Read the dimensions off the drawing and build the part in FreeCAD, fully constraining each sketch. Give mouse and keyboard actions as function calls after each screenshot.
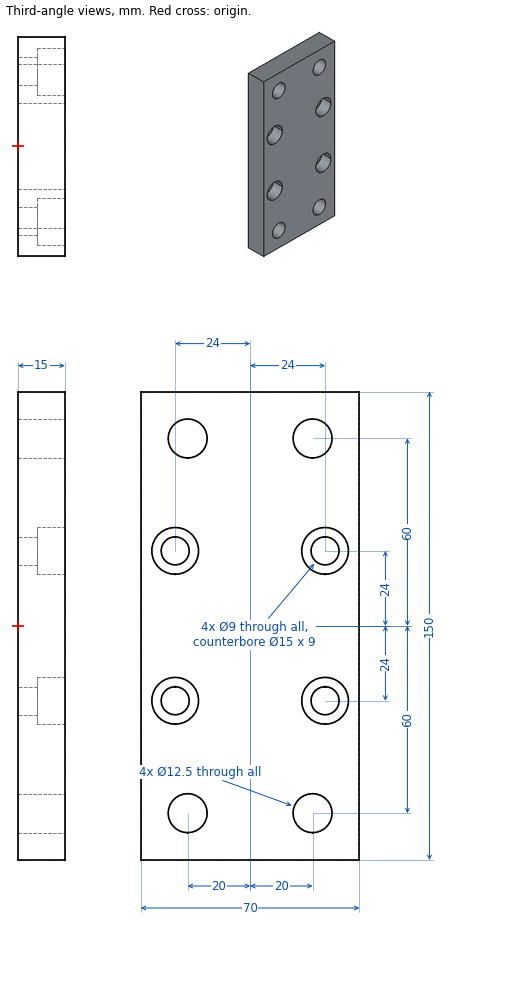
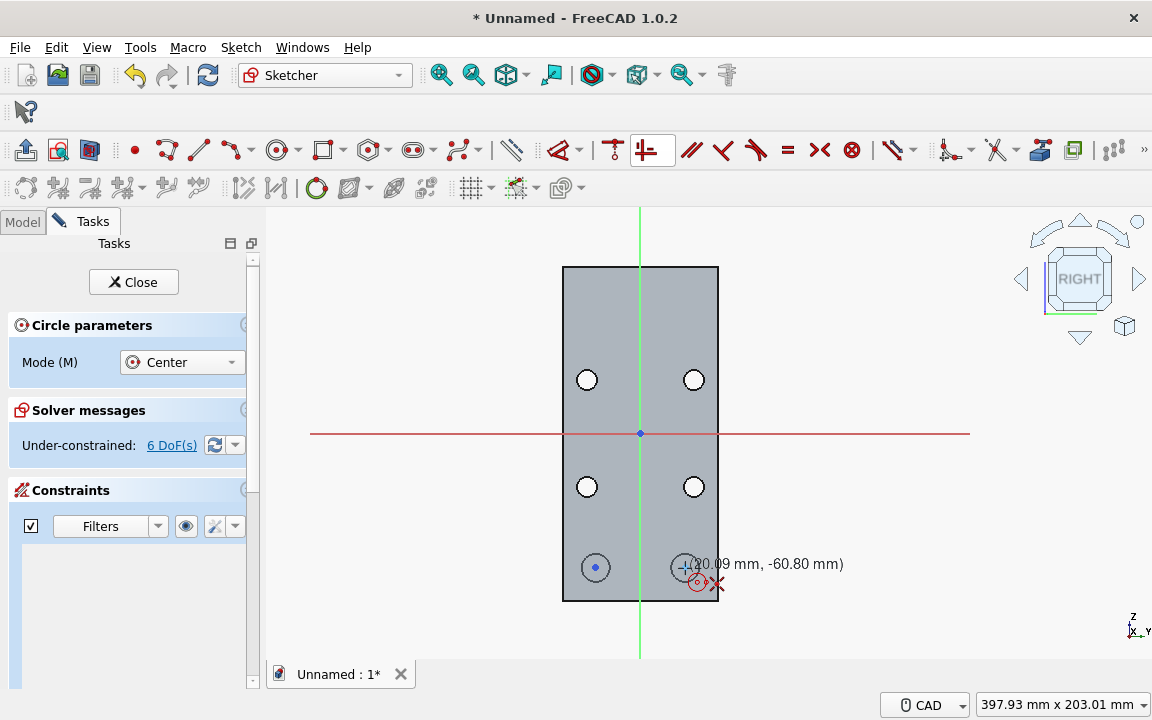
scroll(685, 300, up, 3)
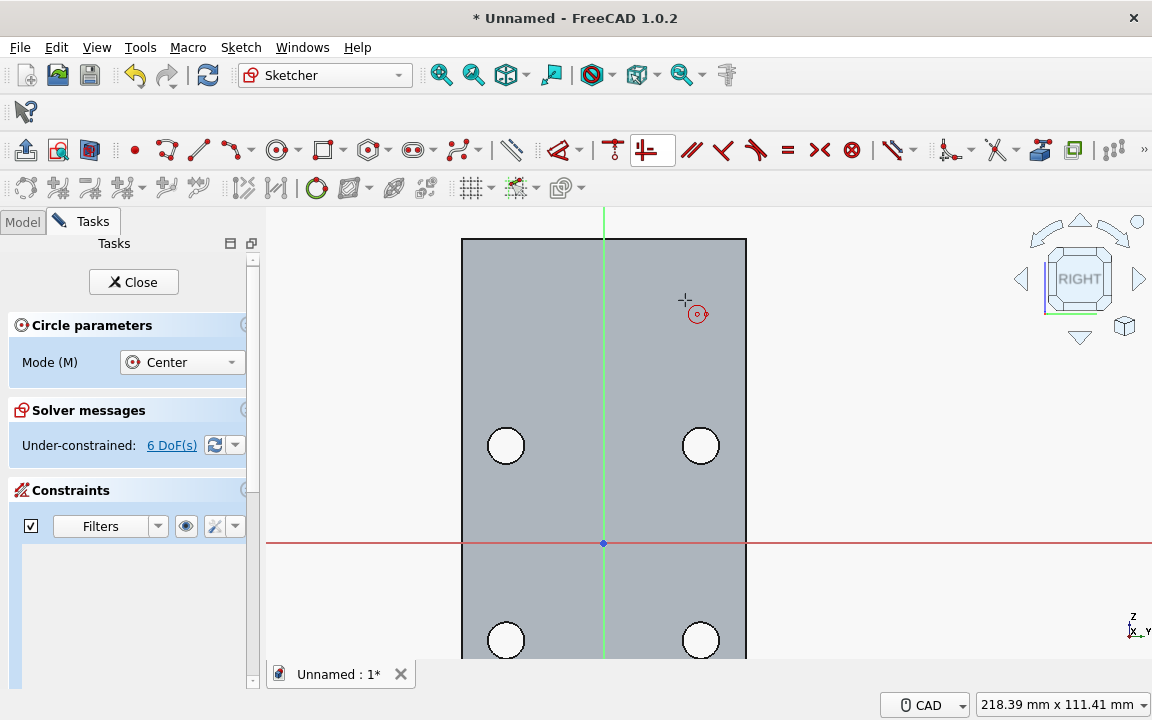
click(685, 300)
click(703, 282)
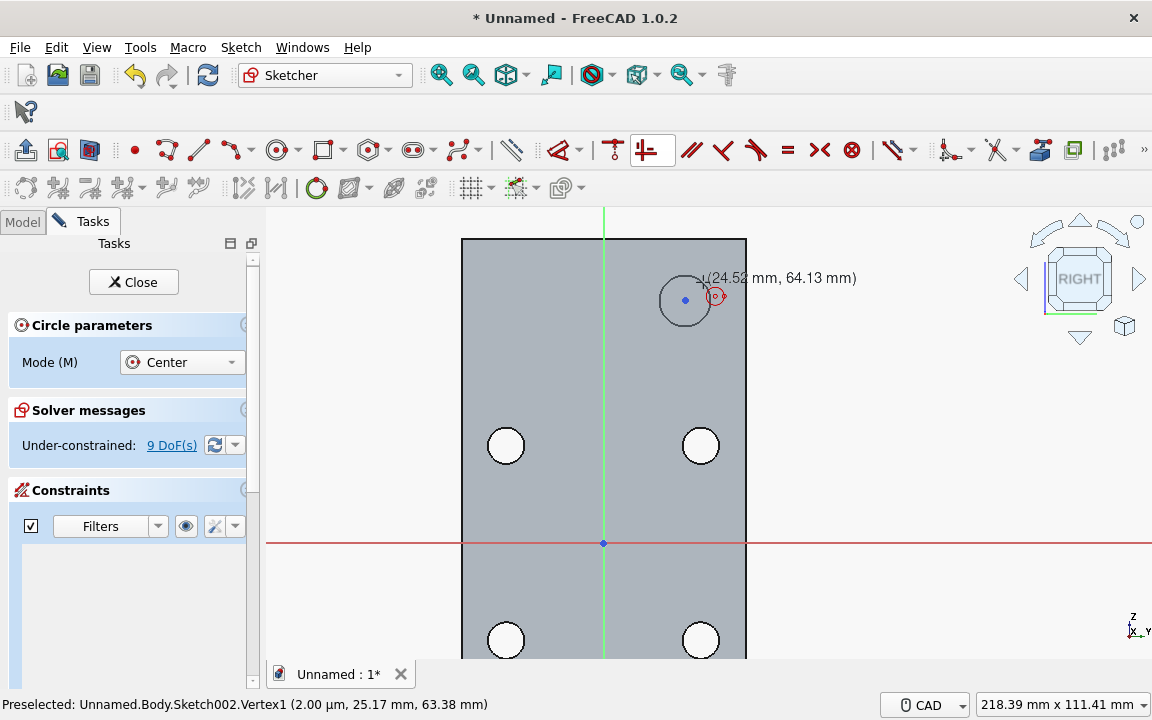
click(522, 300)
click(540, 282)
key(Escape)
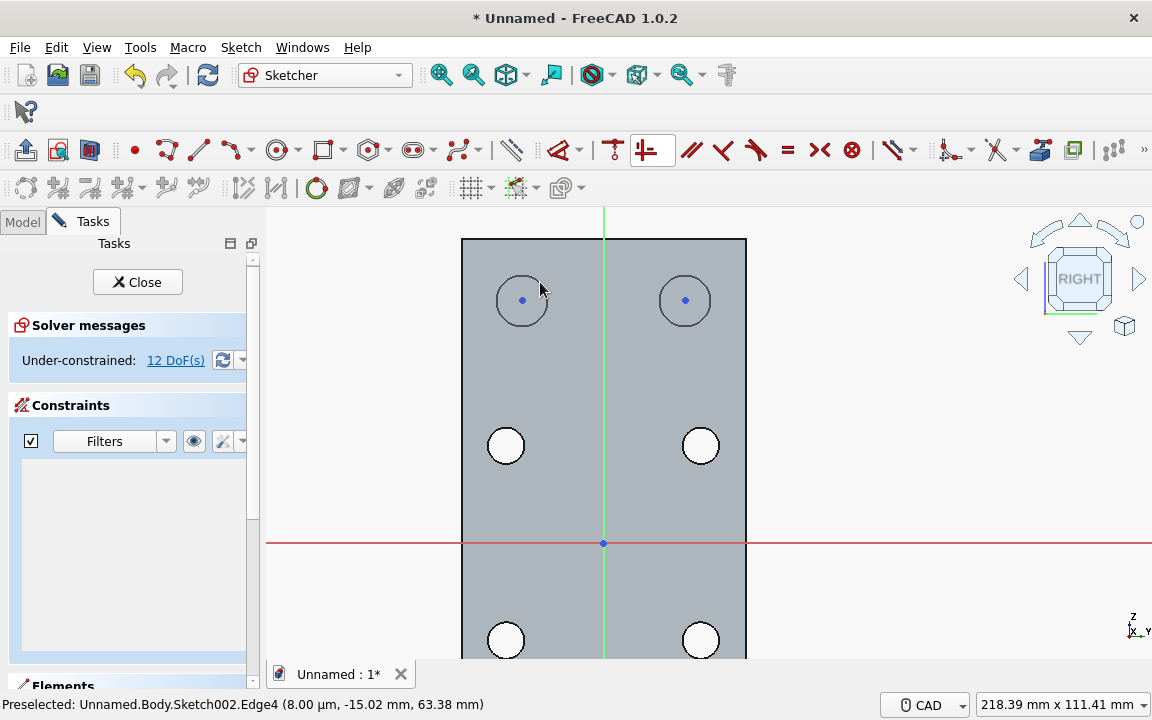
scroll(685, 299, down, 3)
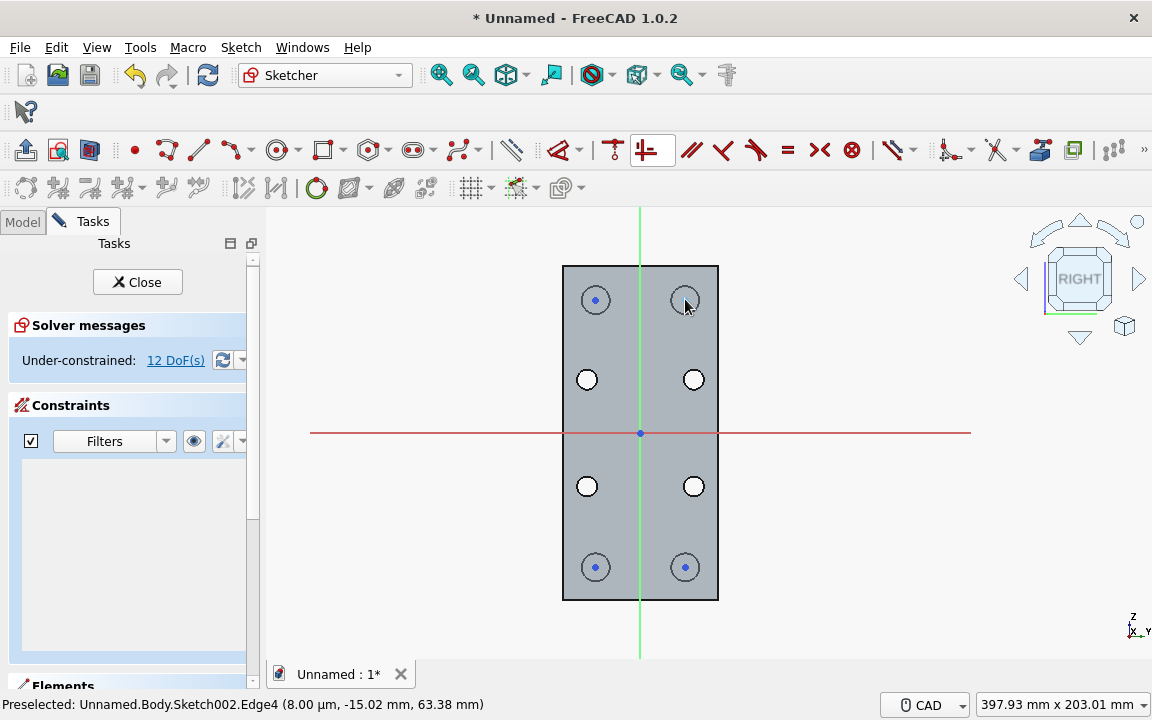
click(695, 557)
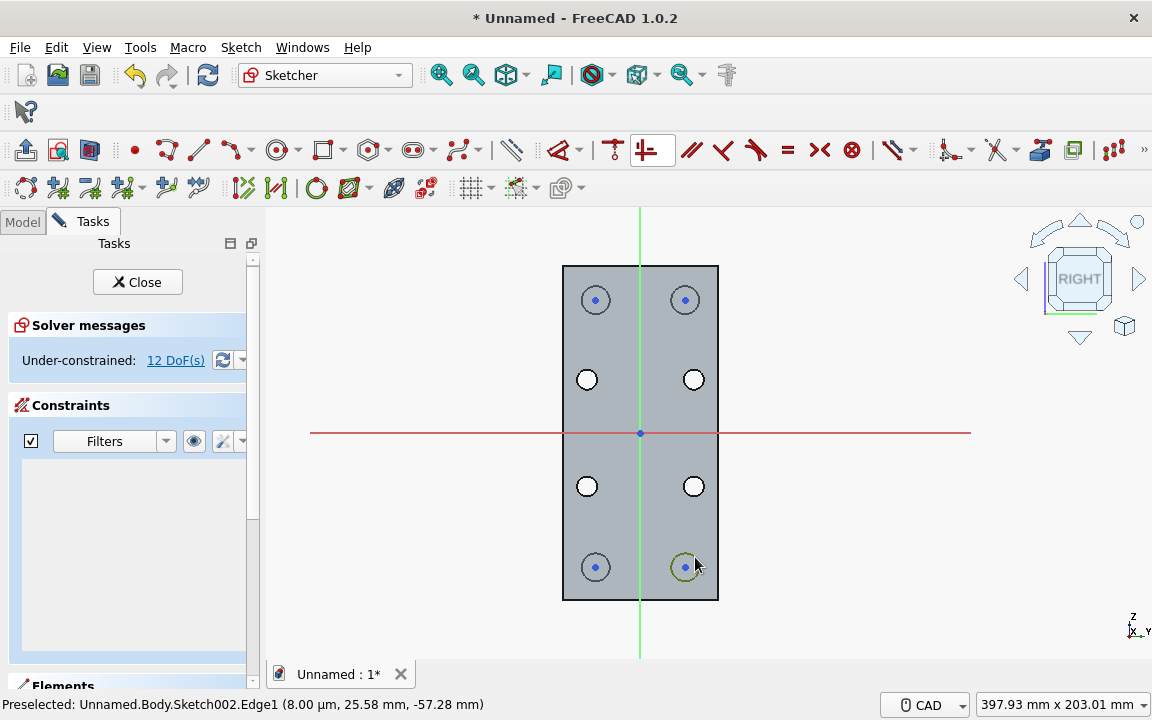
click(606, 557)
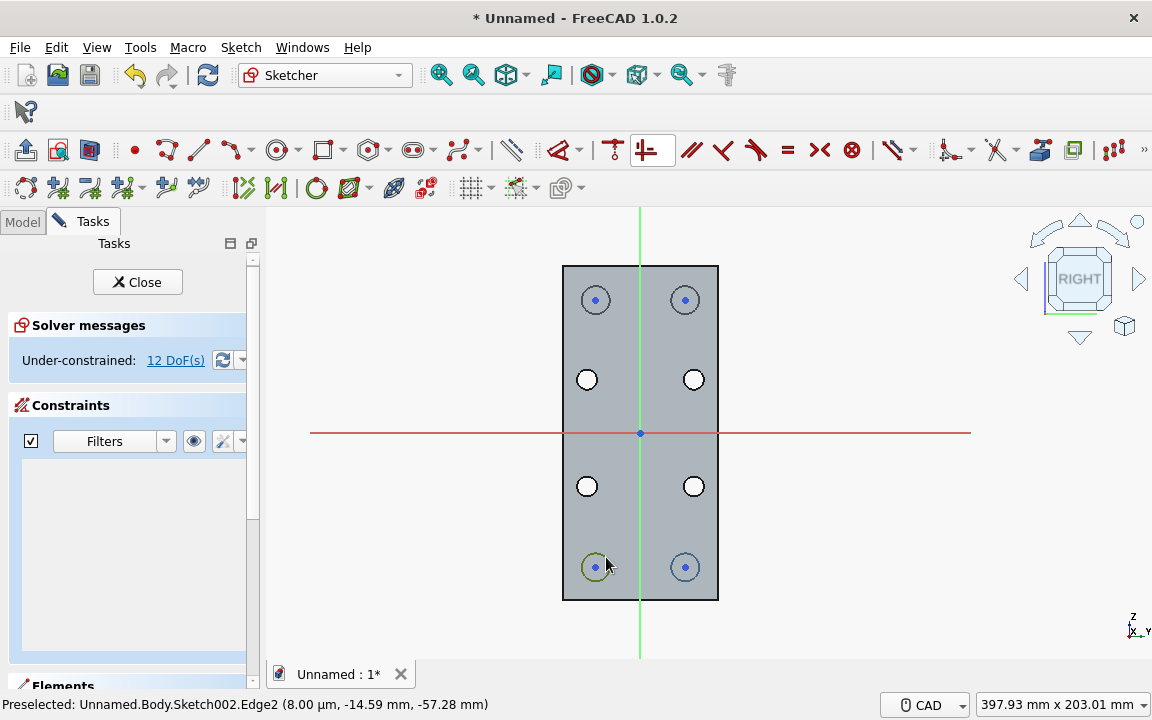
click(695, 290)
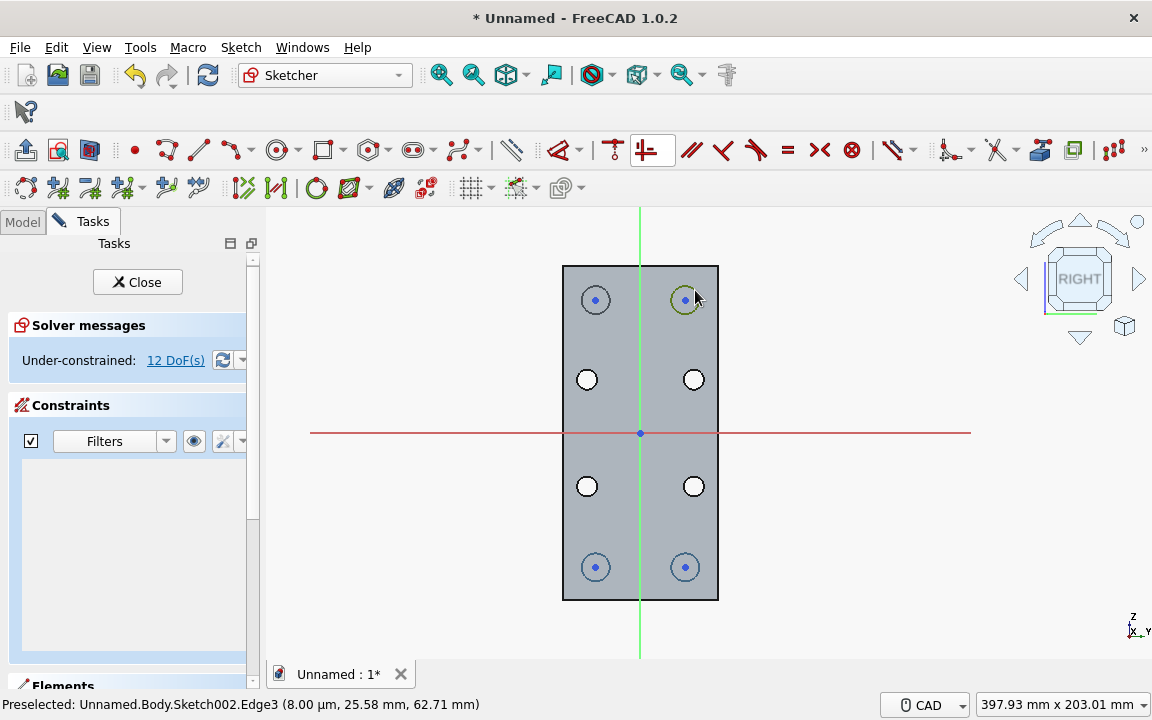
click(606, 290)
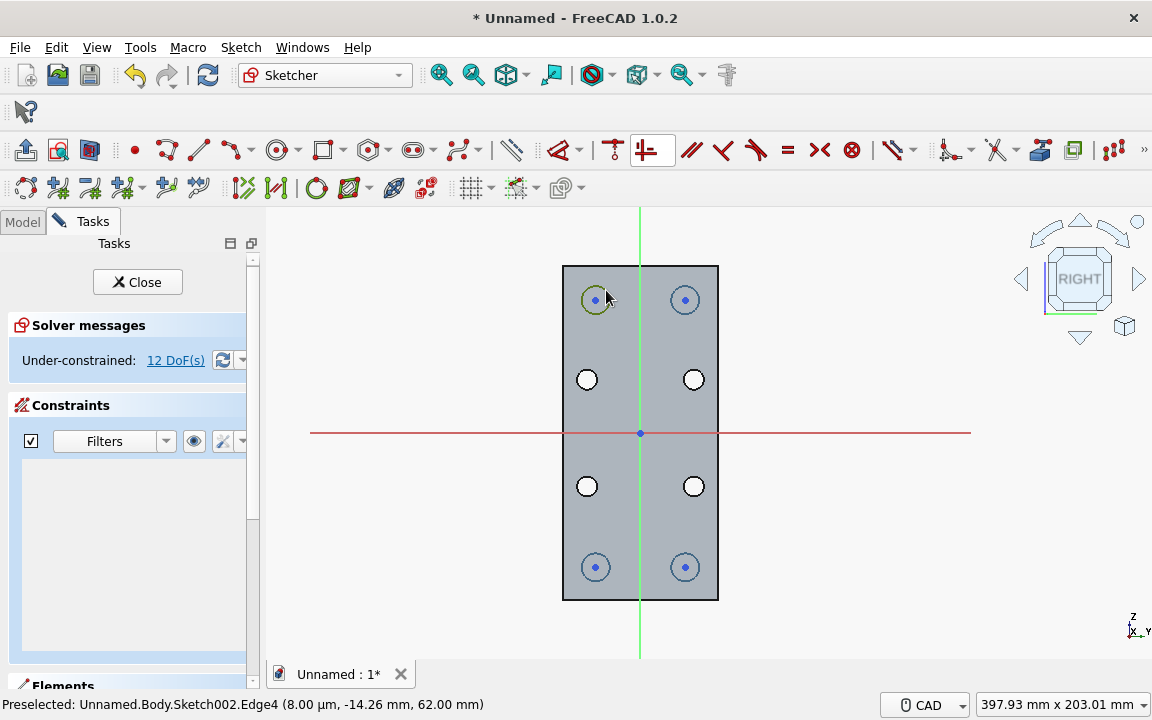
click(788, 150)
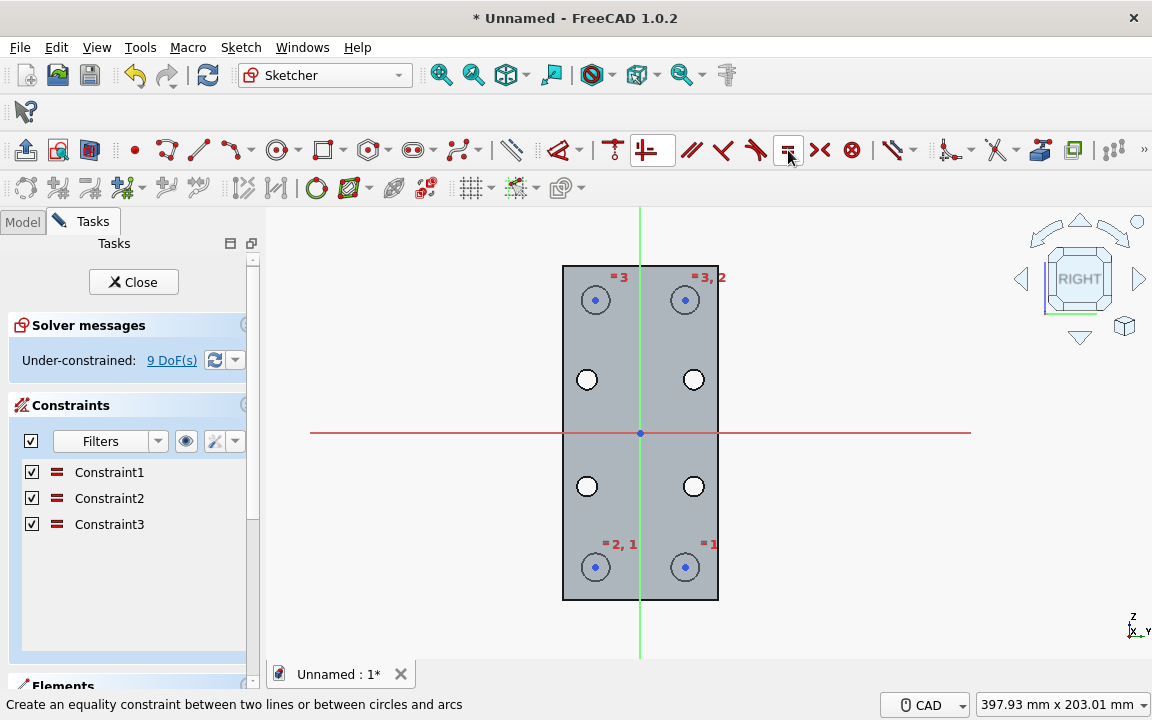
click(685, 567)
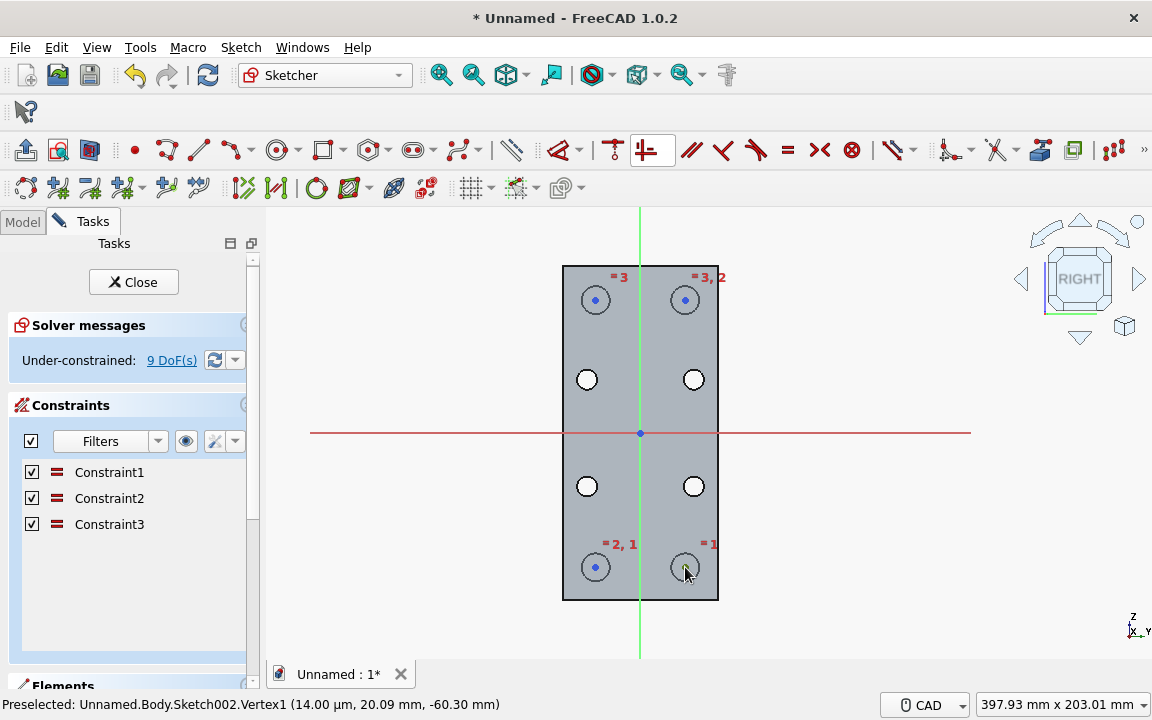
click(596, 567)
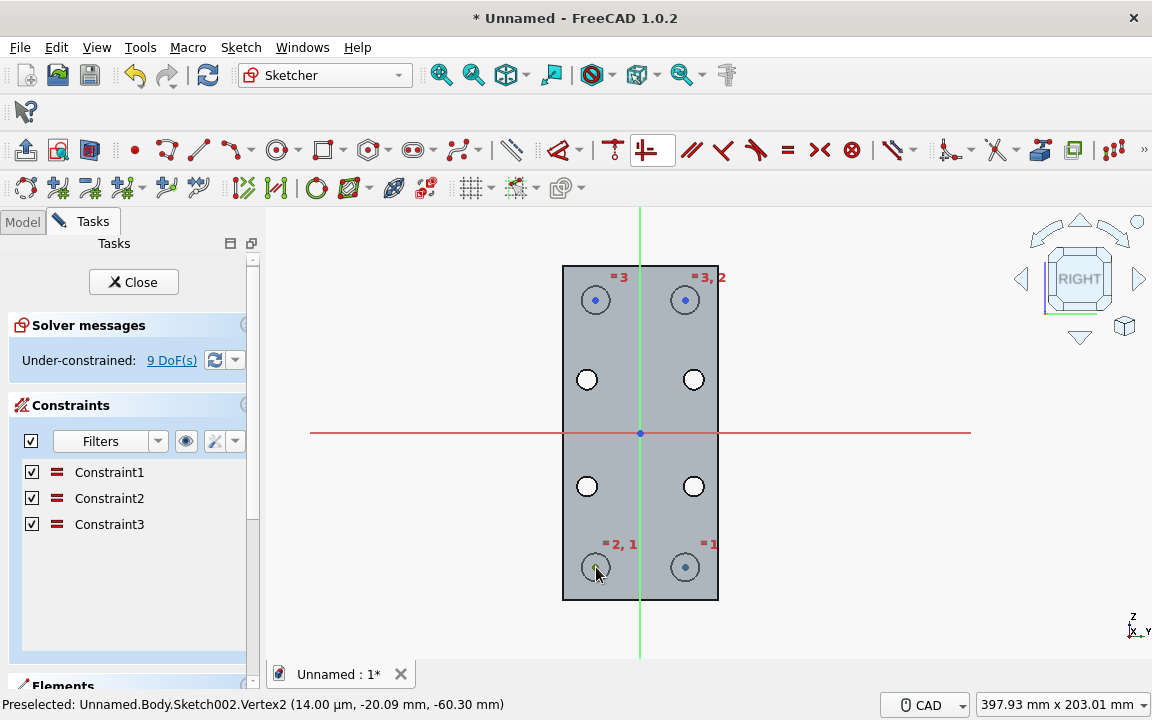
click(670, 150)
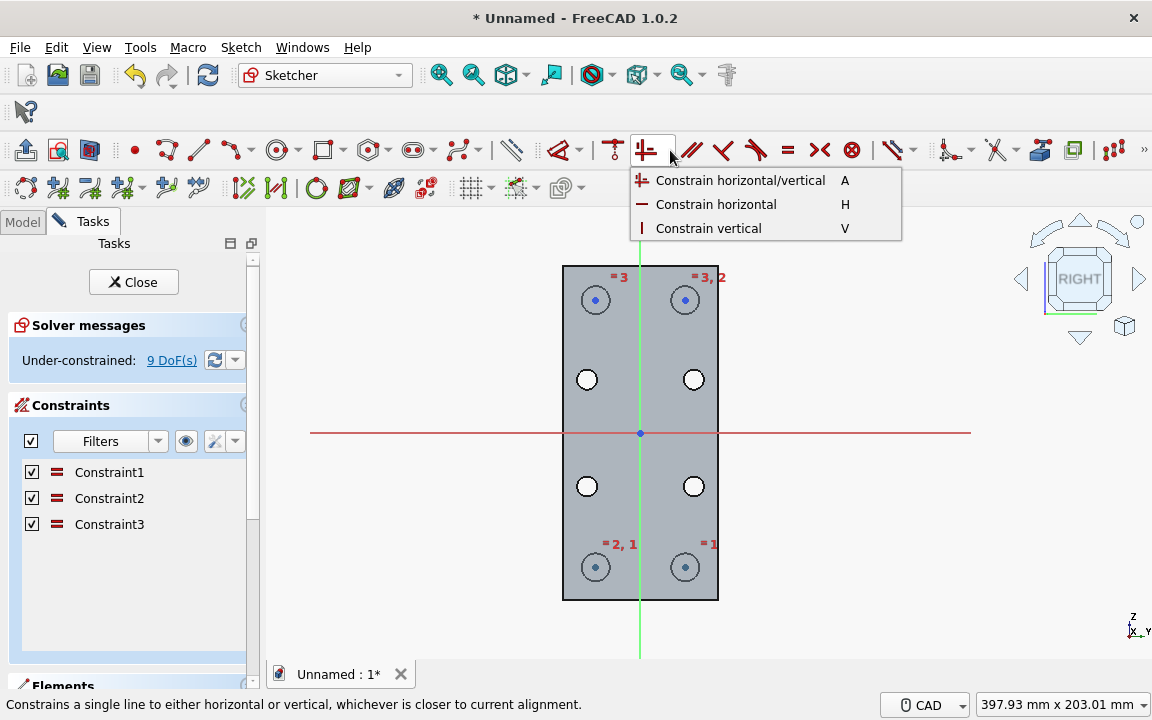
click(766, 204)